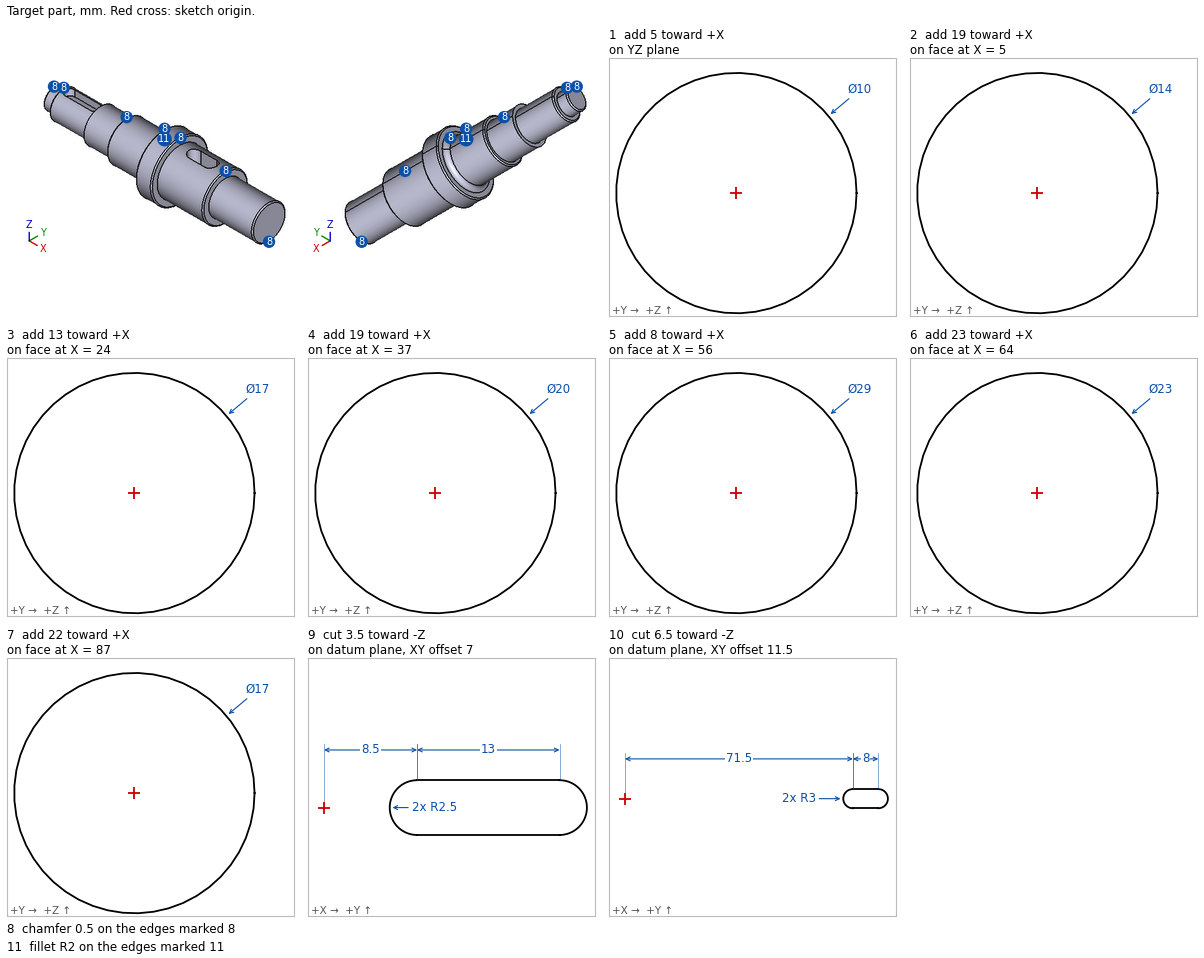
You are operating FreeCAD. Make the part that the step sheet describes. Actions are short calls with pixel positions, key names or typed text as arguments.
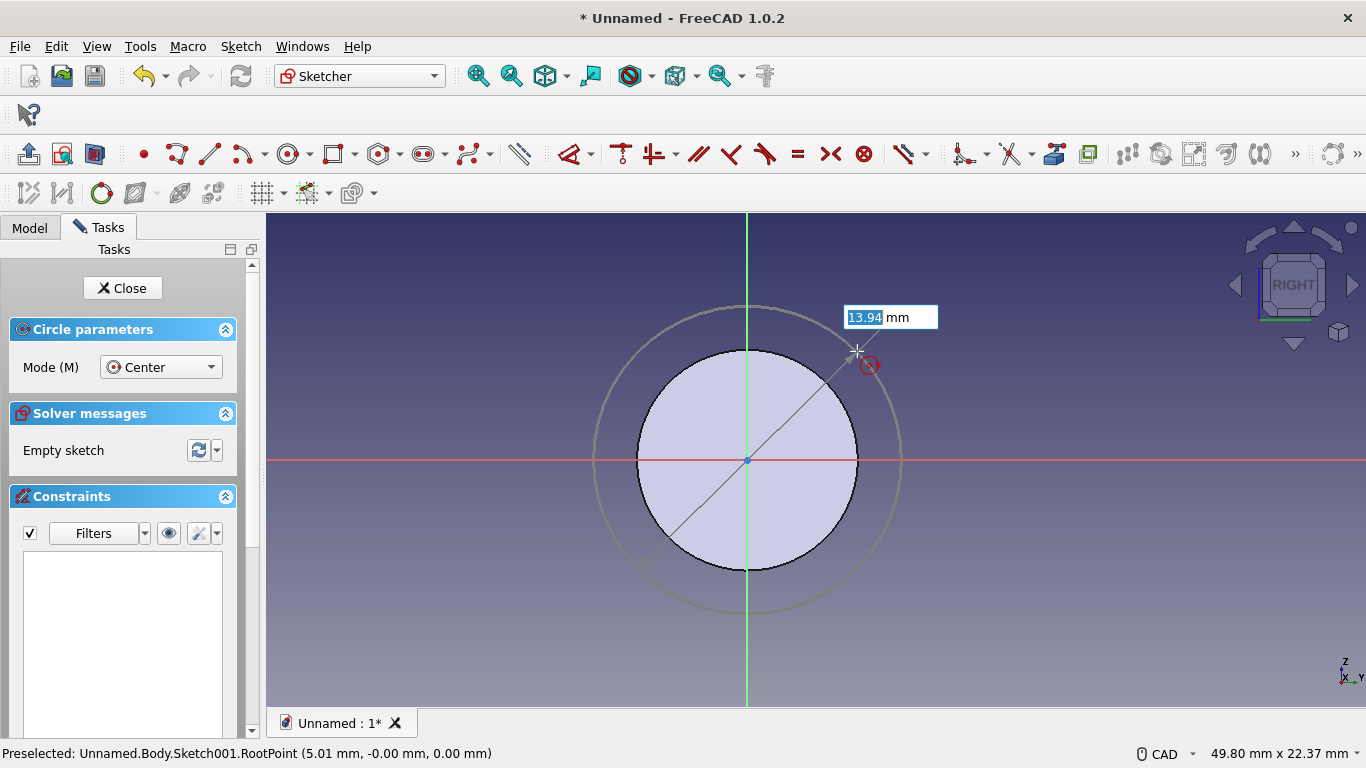
text(14)
key(Return)
key(Escape)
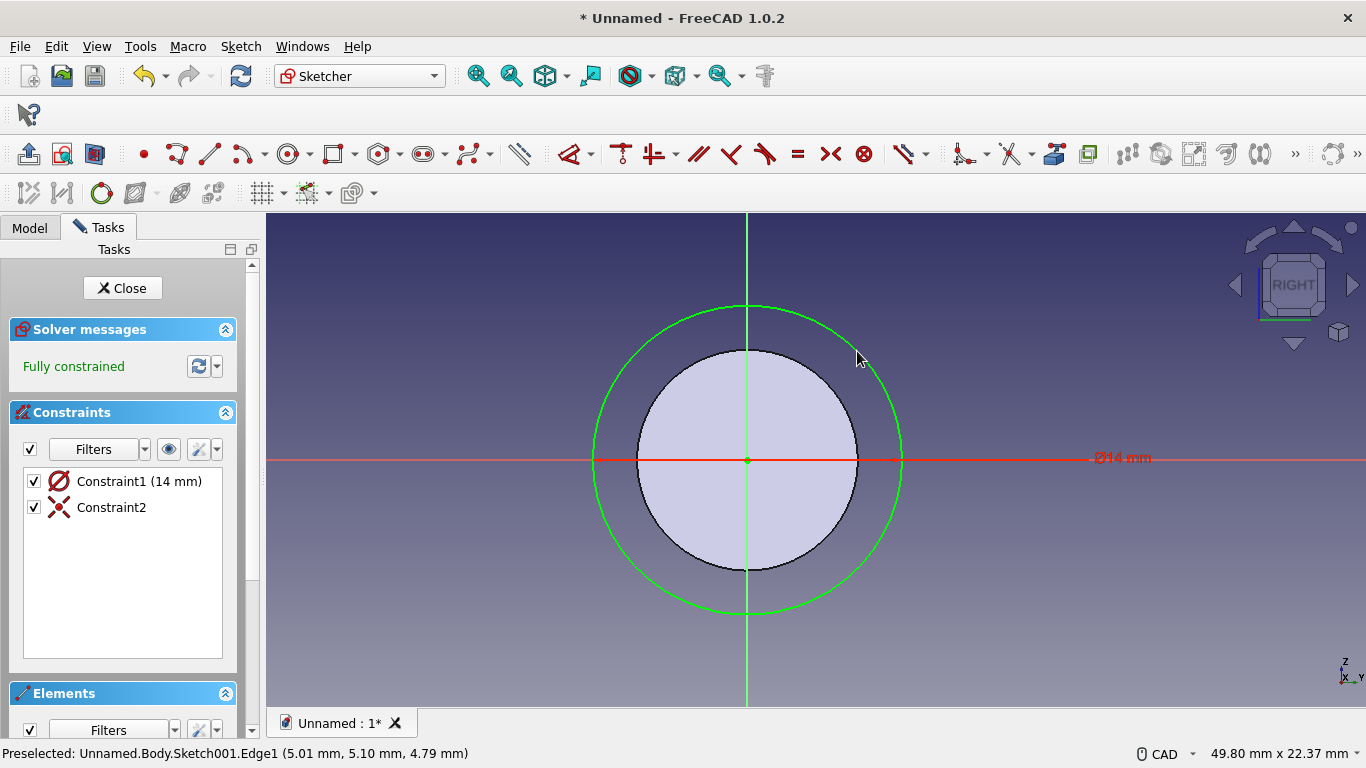
click(123, 288)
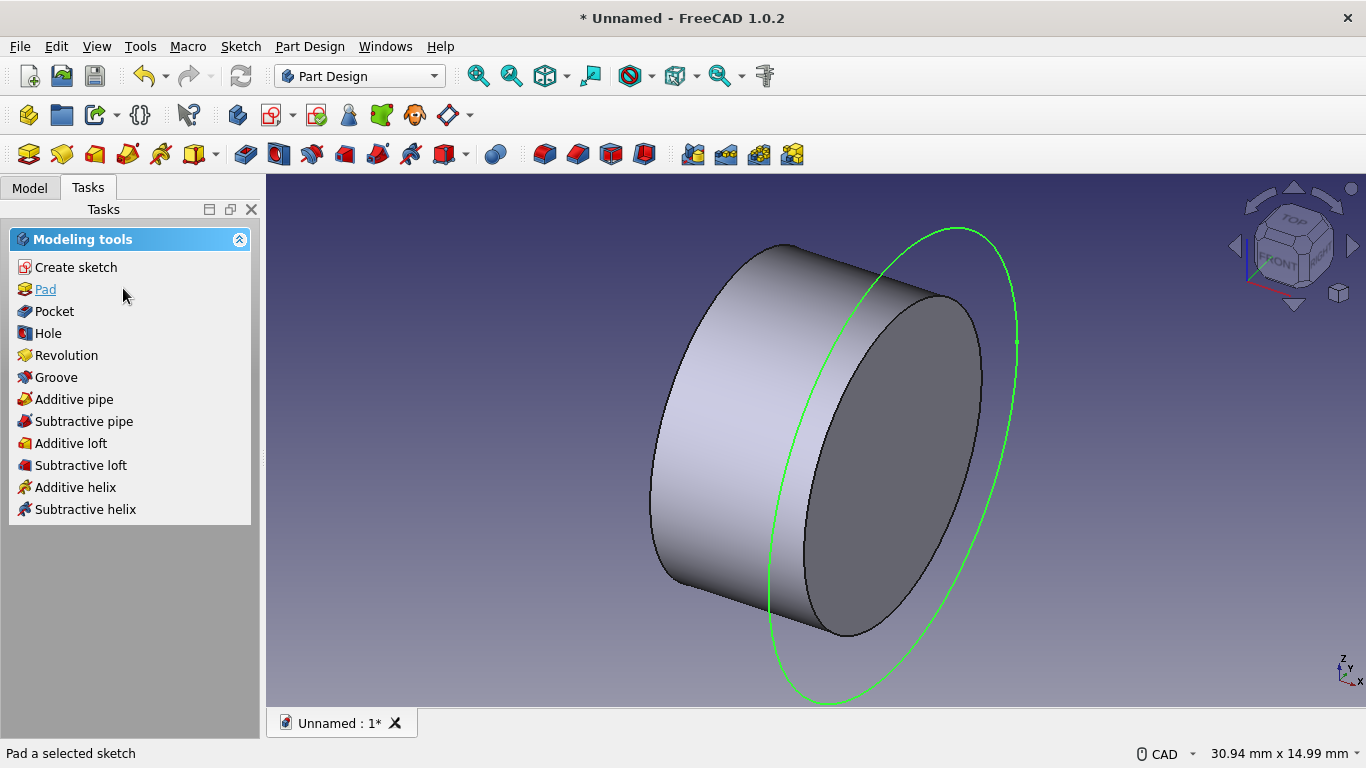
click(29, 154)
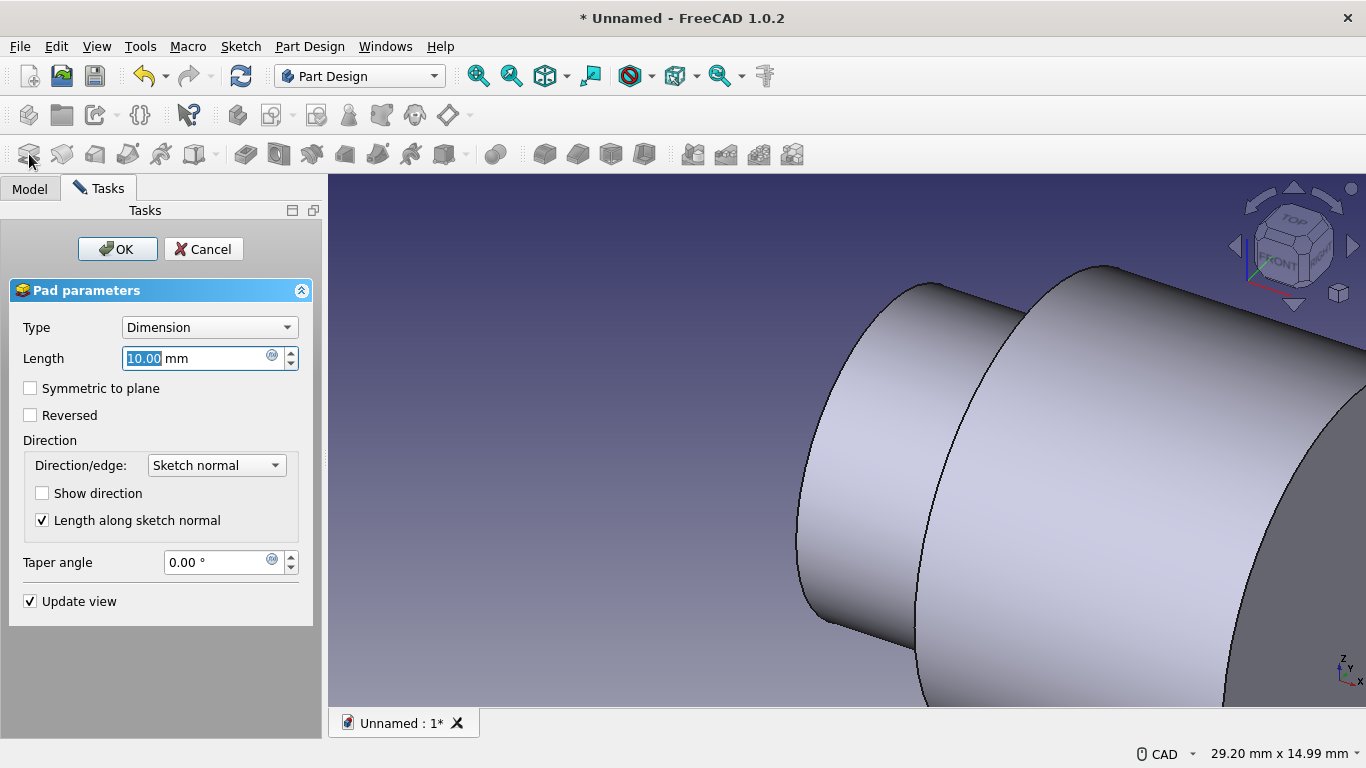
text(19)
key(Tab)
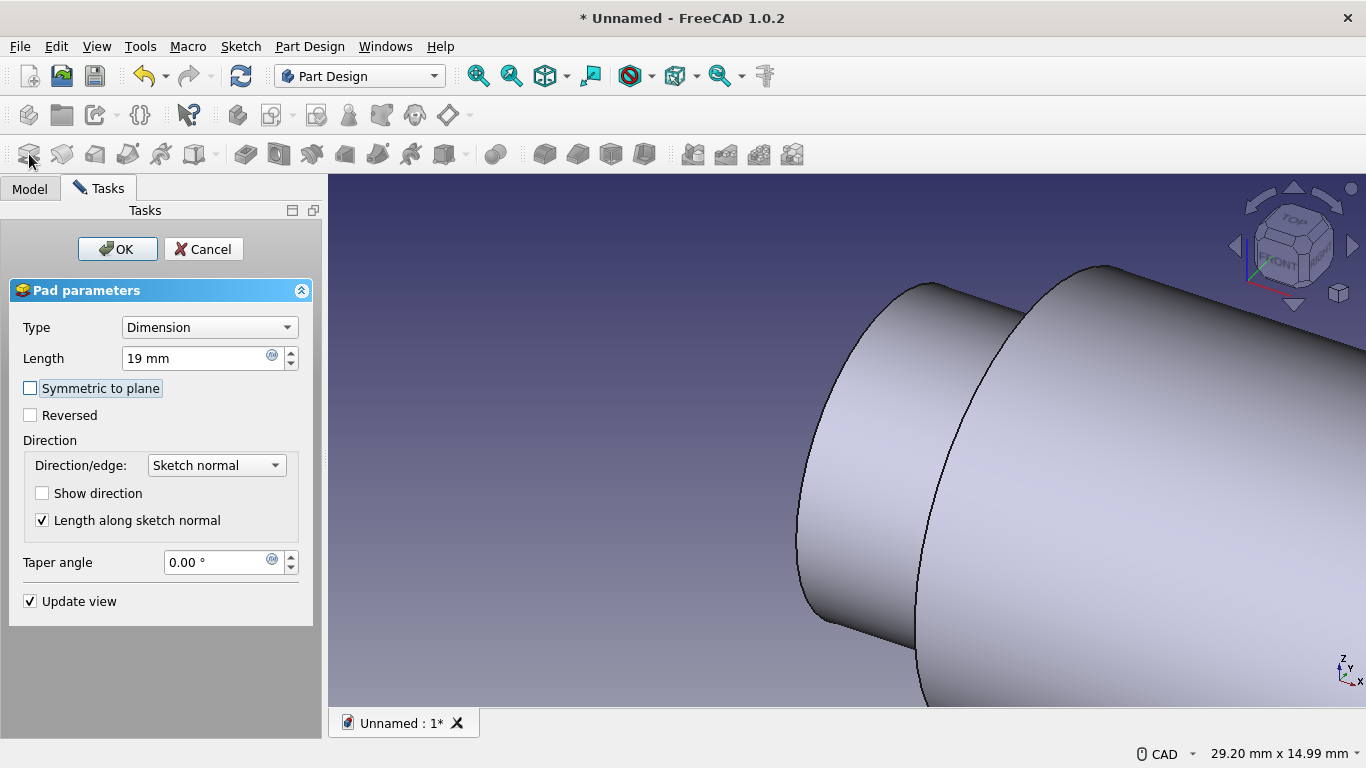
click(118, 249)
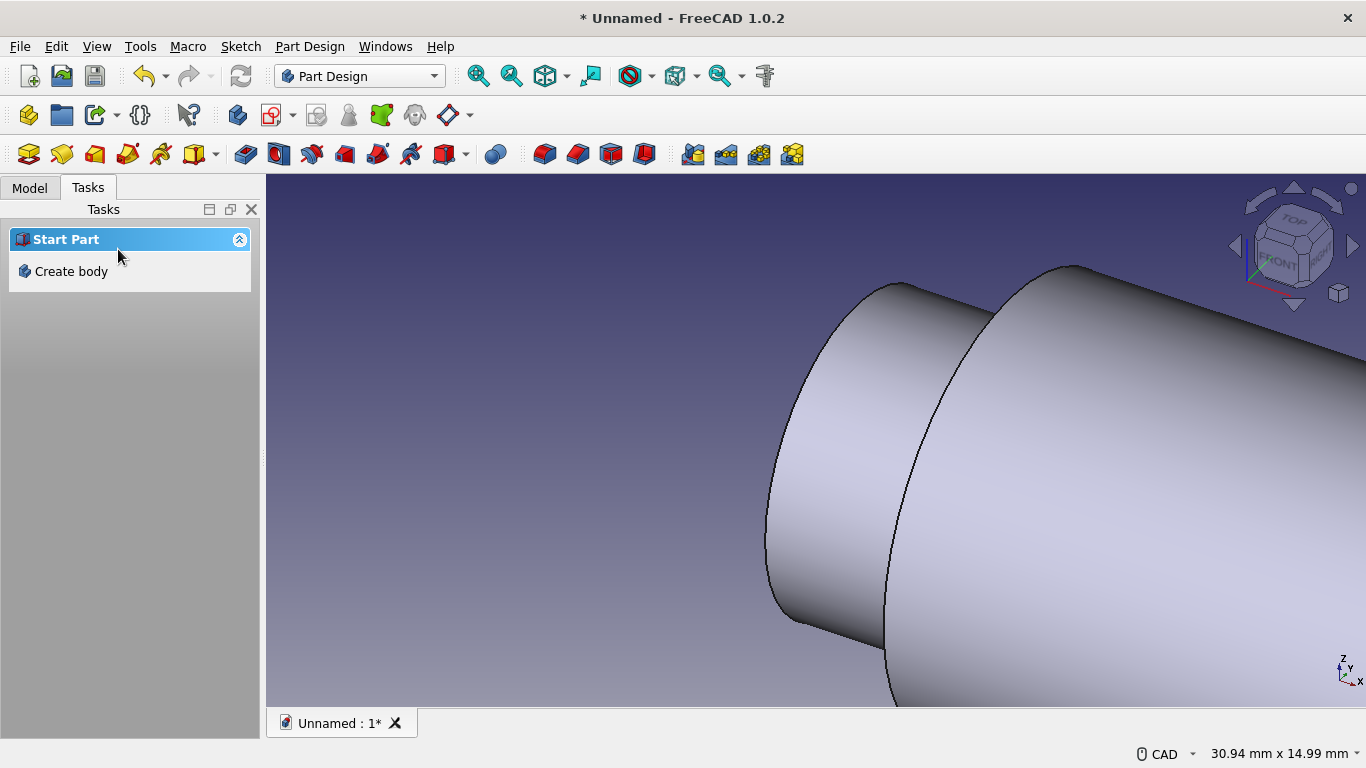
click(479, 76)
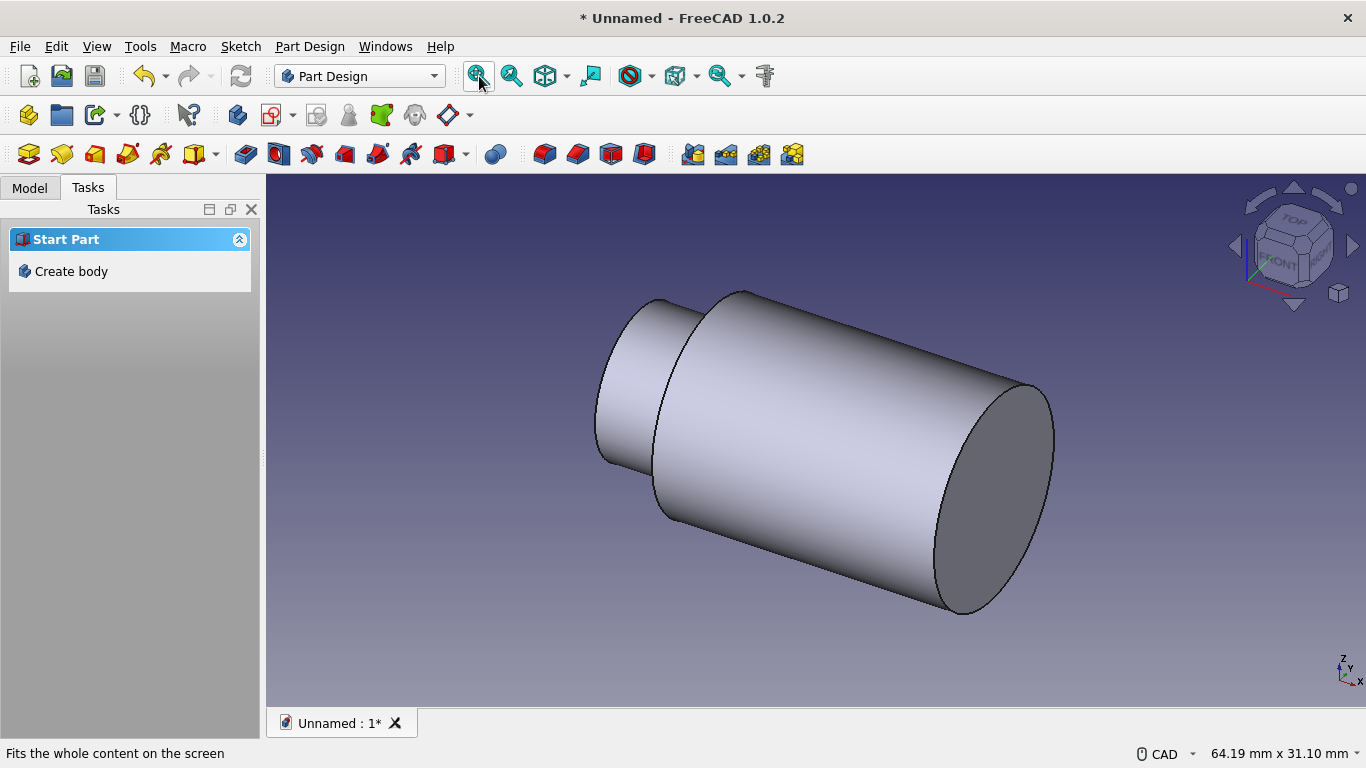
click(994, 499)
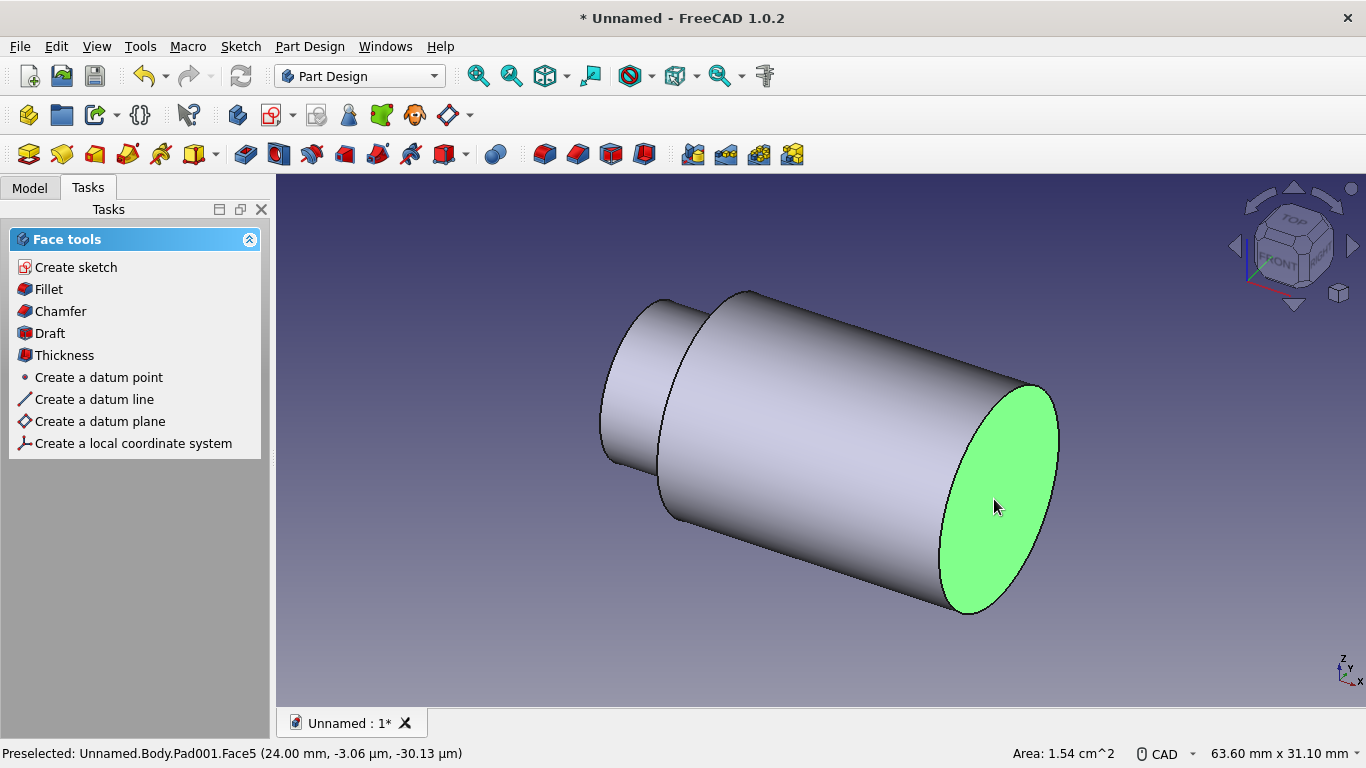
click(270, 116)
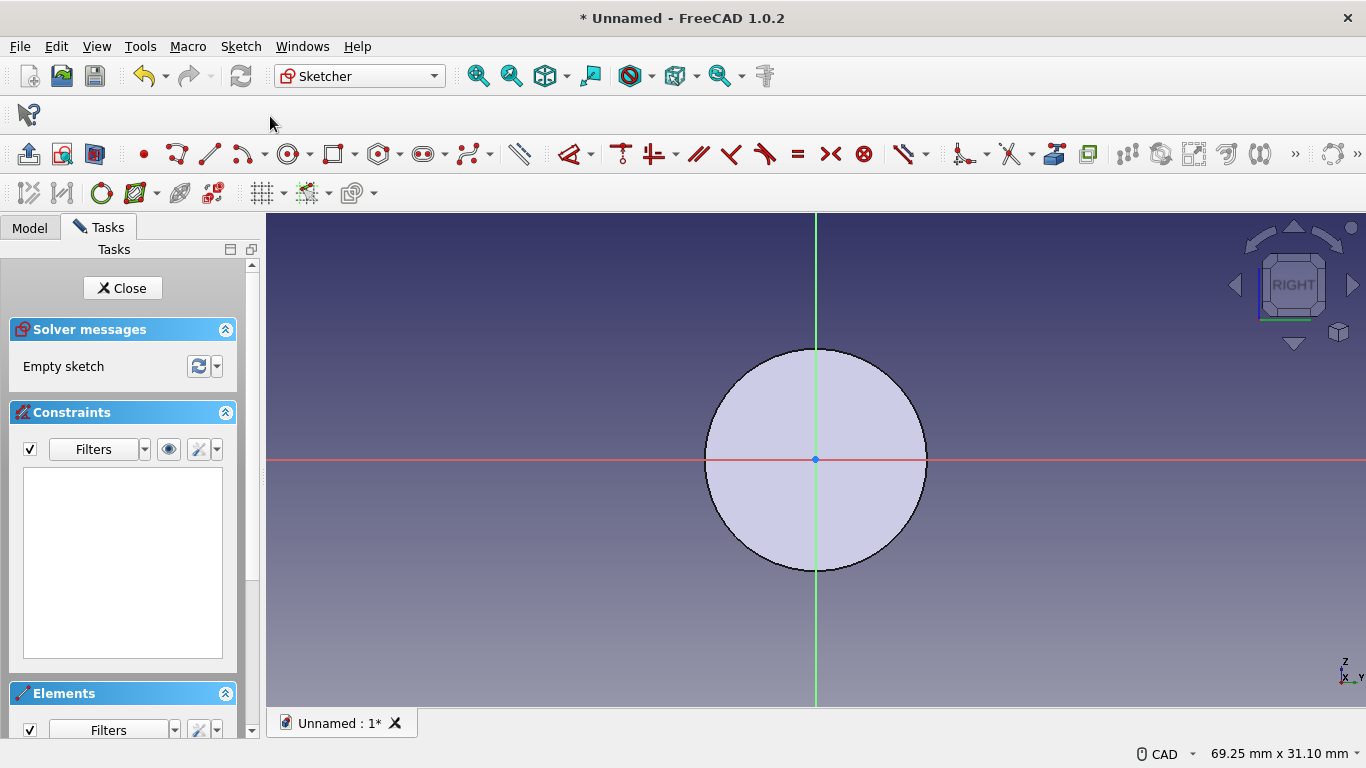
click(288, 154)